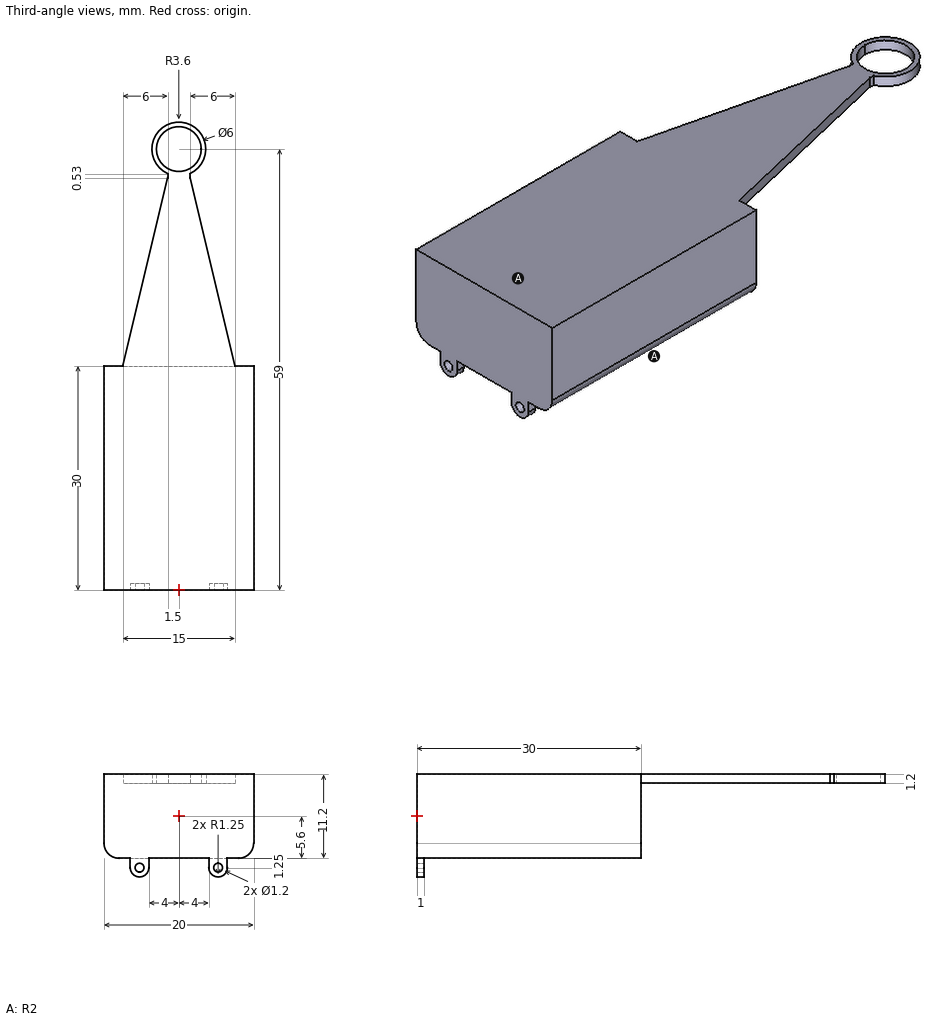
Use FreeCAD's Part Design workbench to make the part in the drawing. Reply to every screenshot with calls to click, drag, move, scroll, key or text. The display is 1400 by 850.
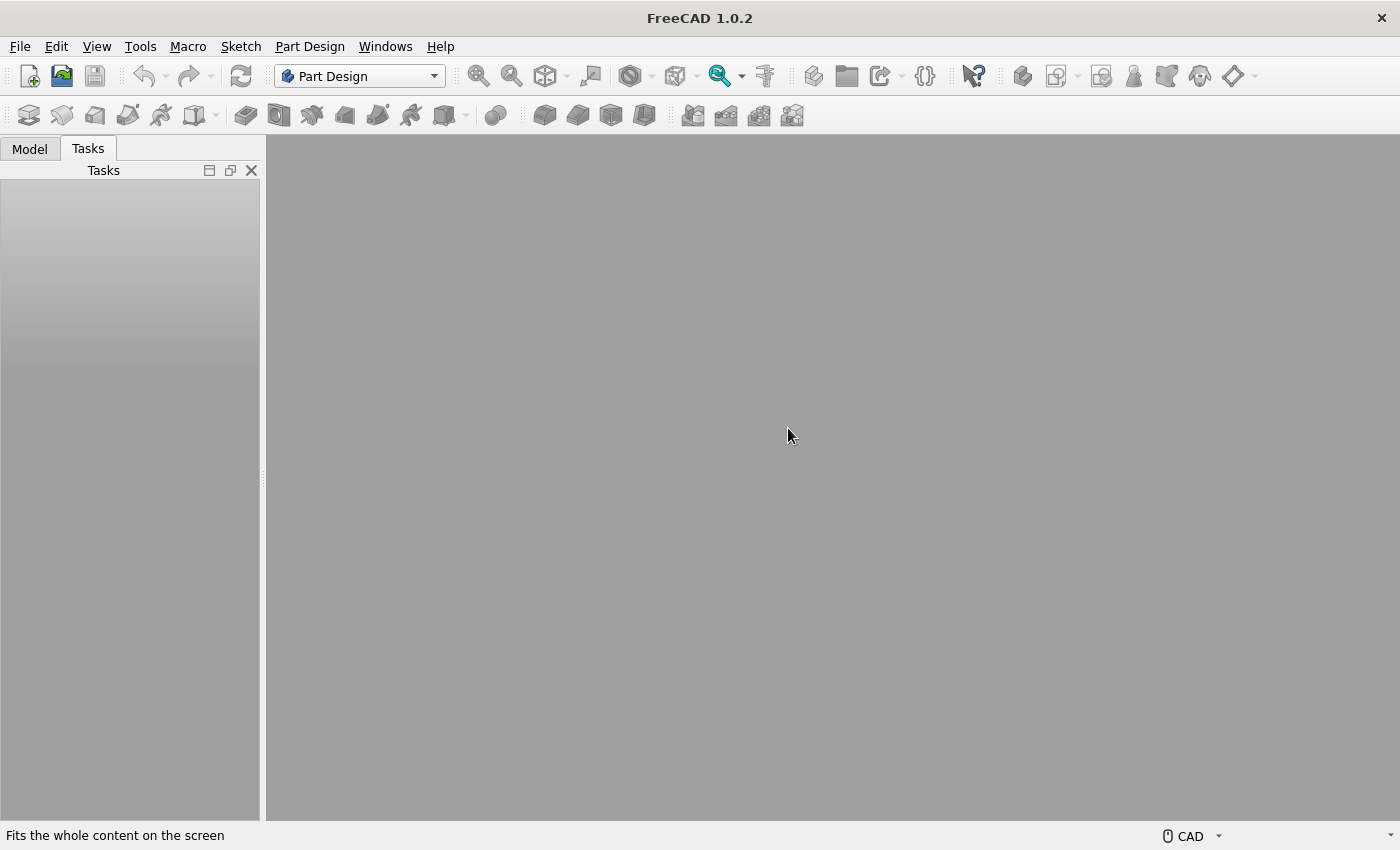
click(29, 76)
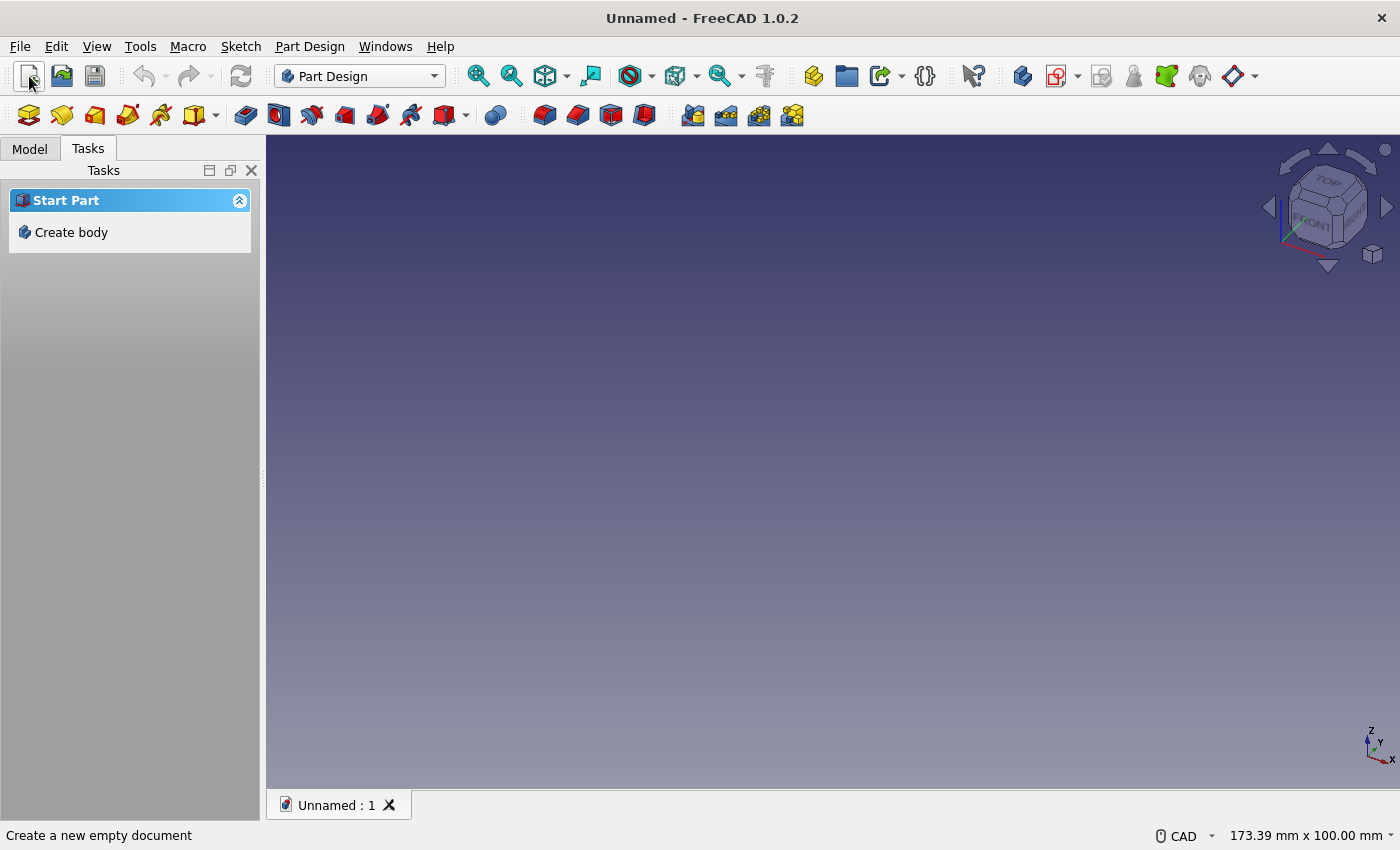
click(1056, 76)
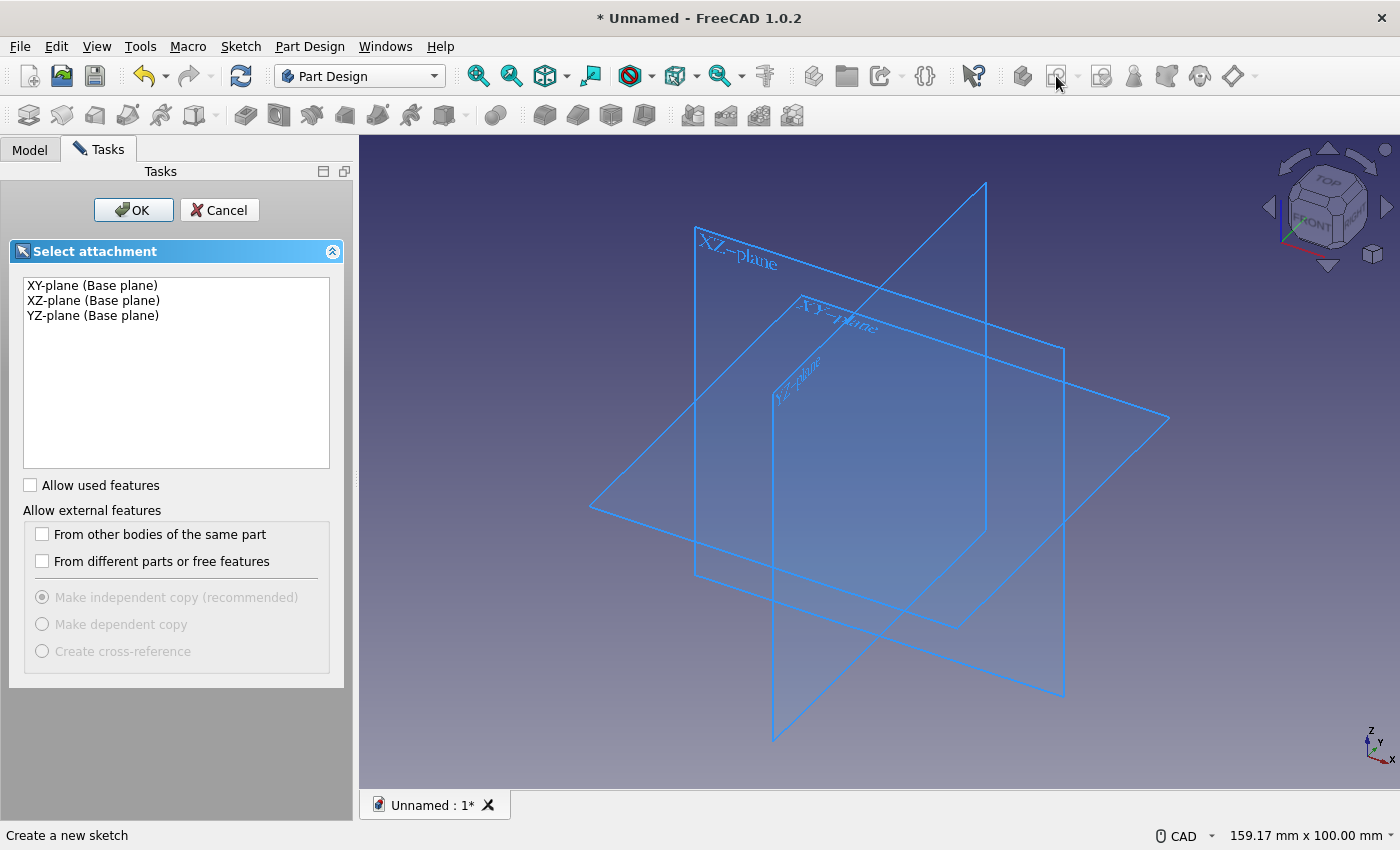
click(84, 300)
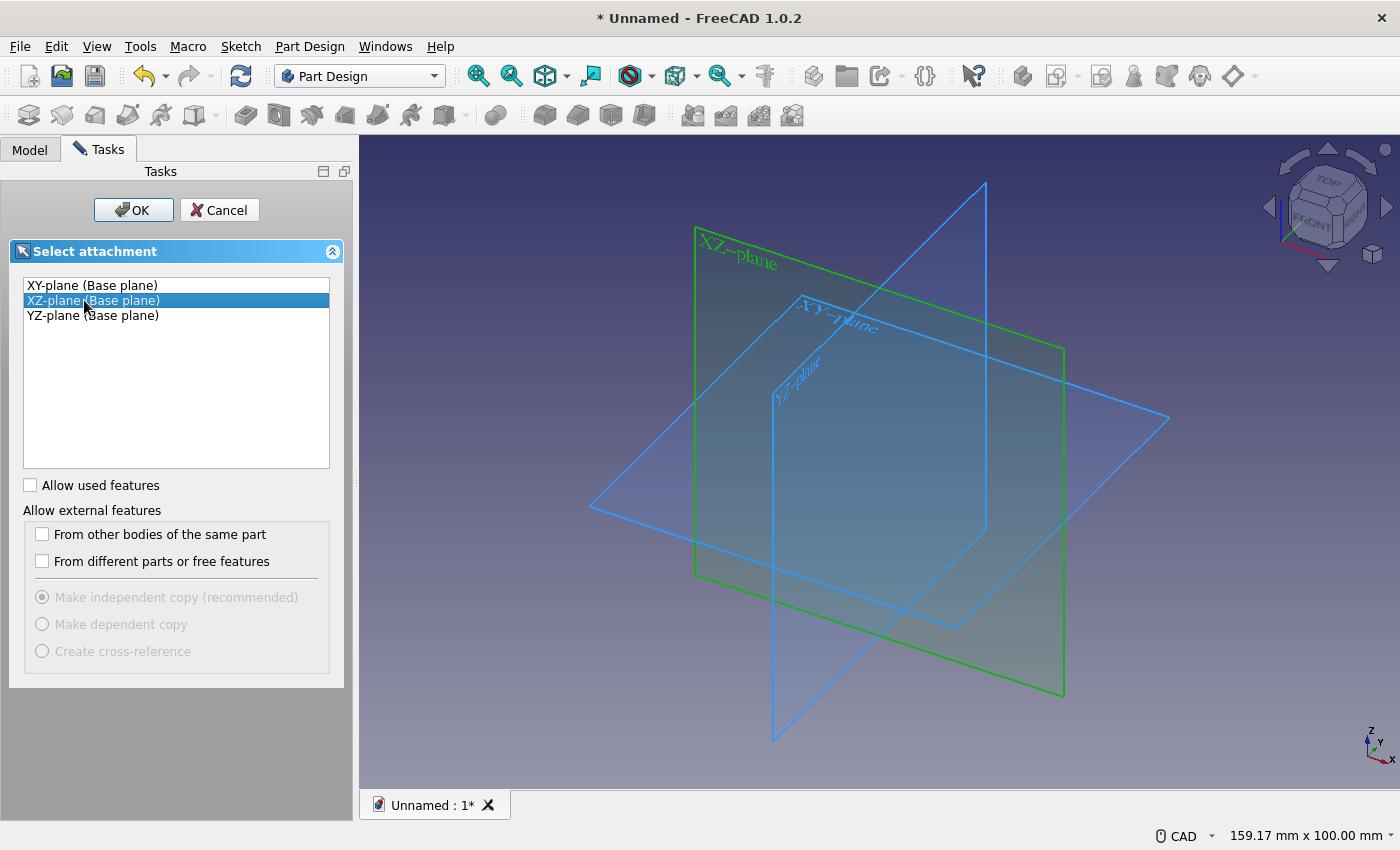
click(134, 210)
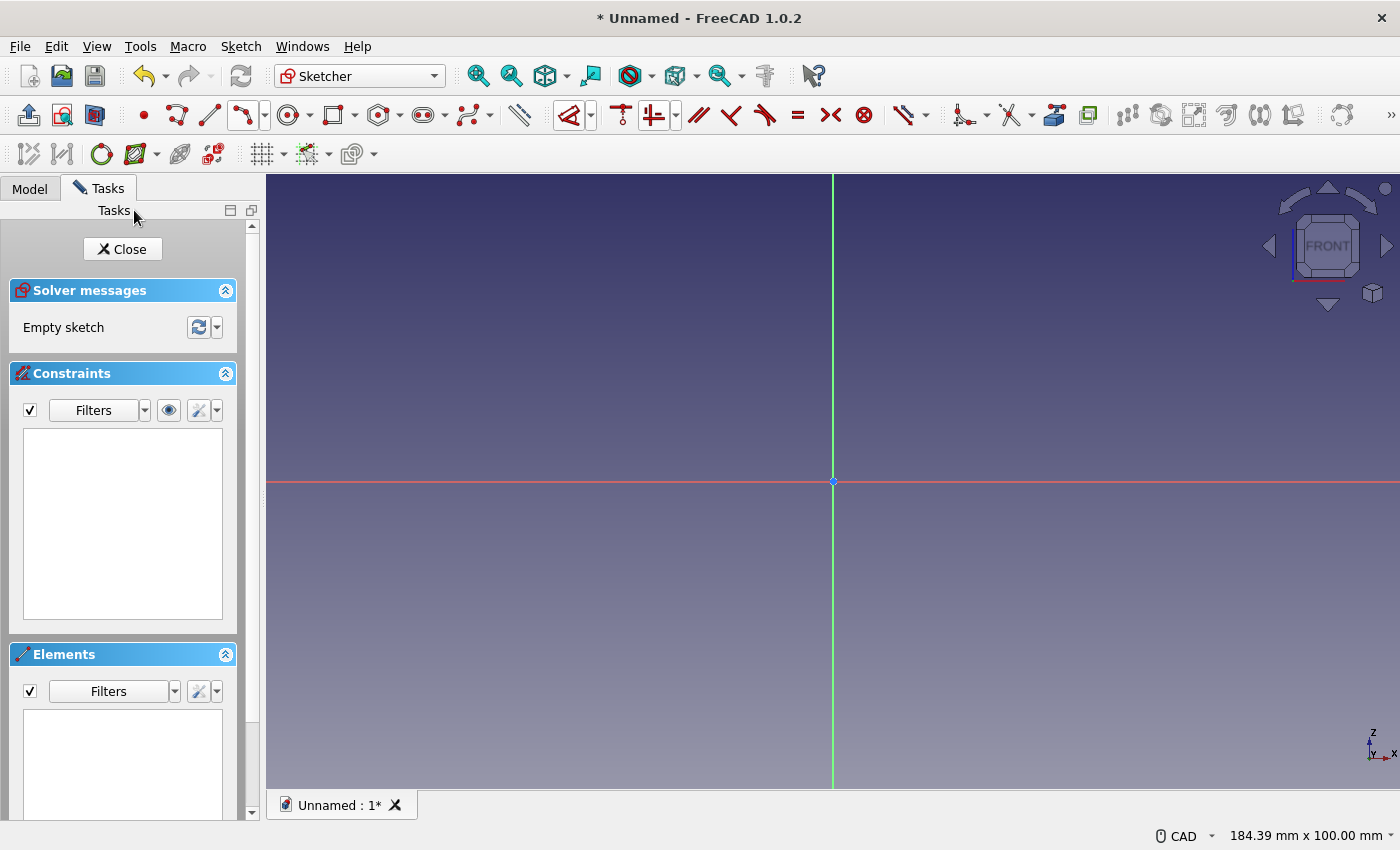
scroll(850, 482, up, 8)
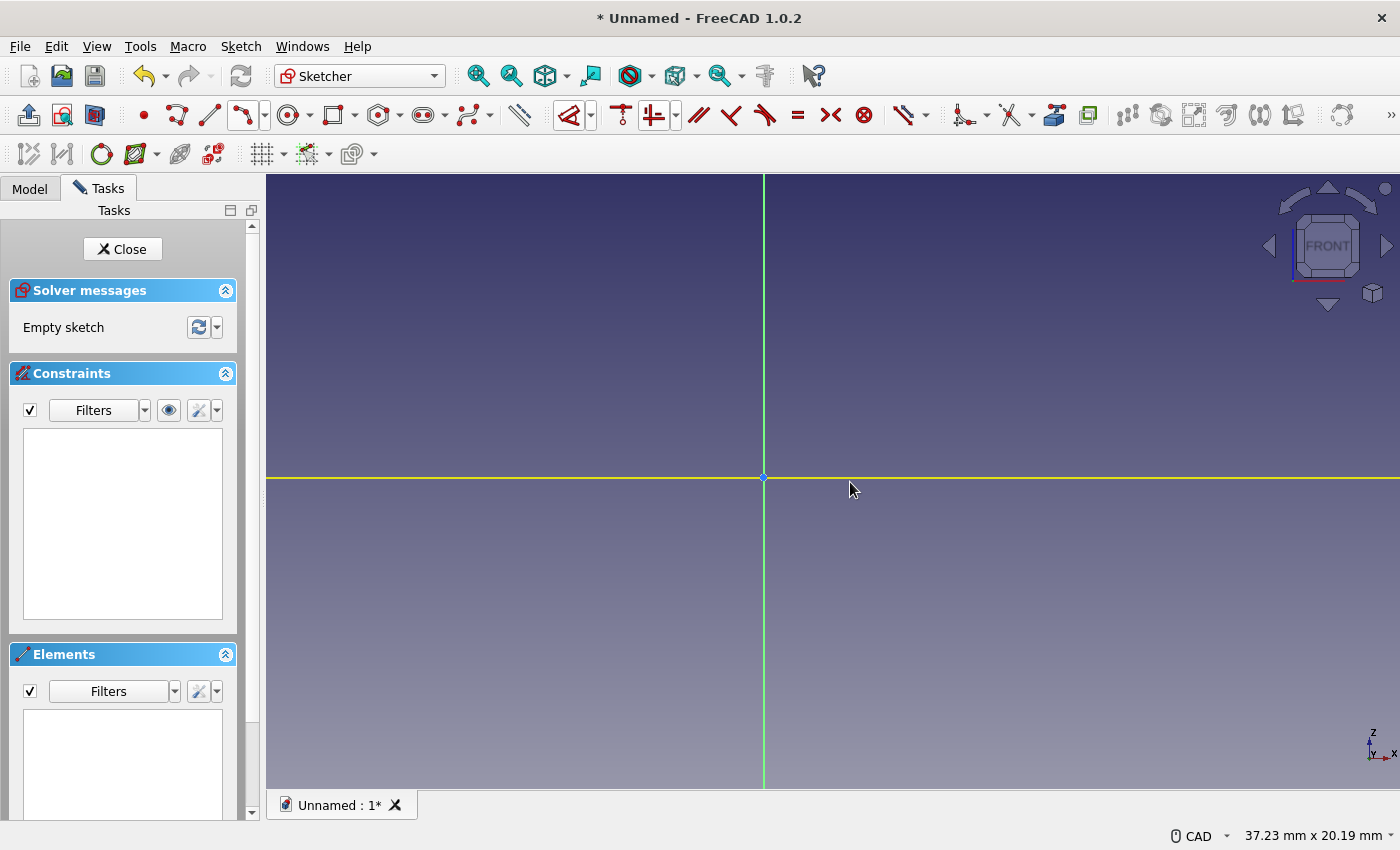
key(g)
key(v)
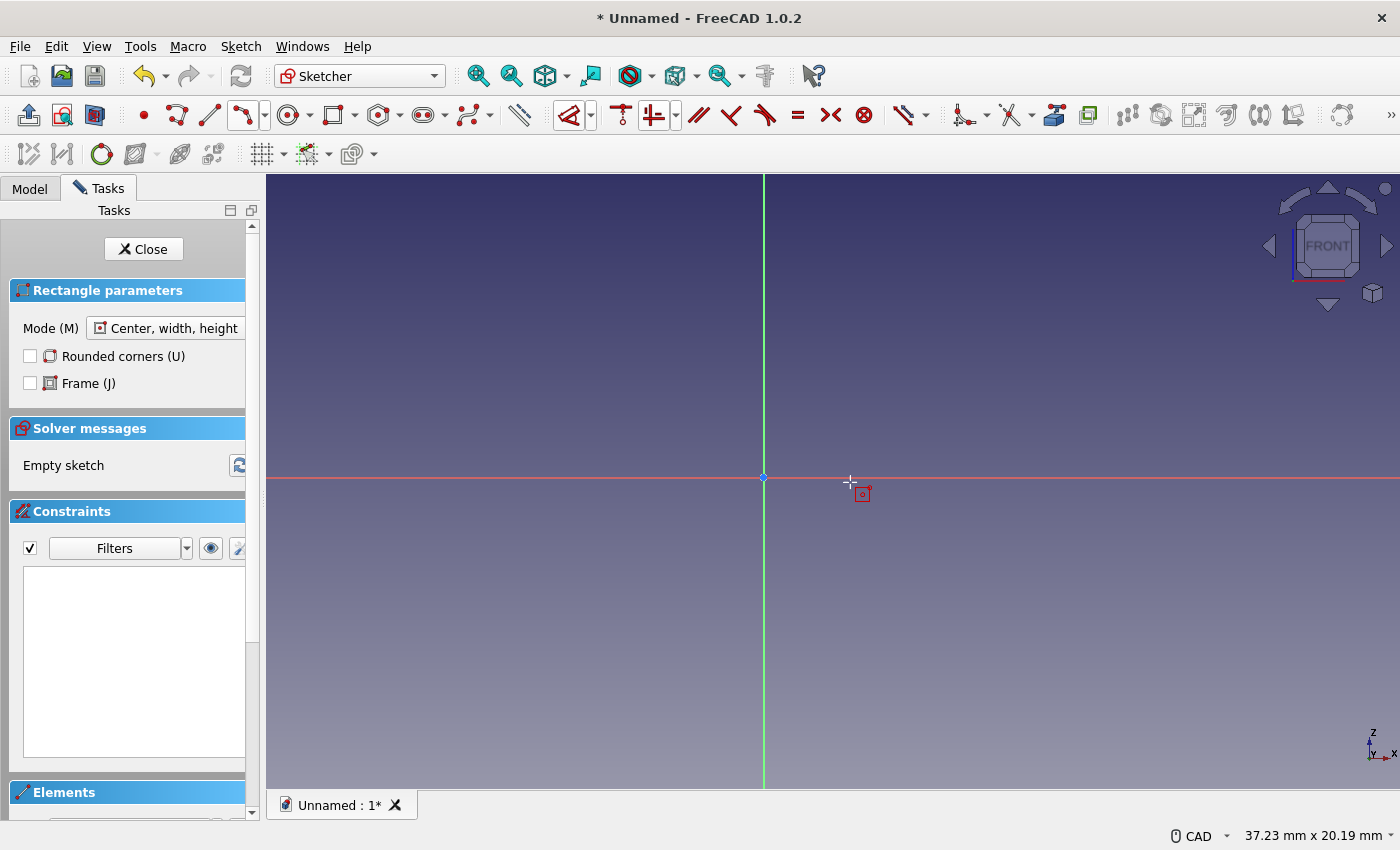
click(764, 478)
click(1068, 307)
key(Escape)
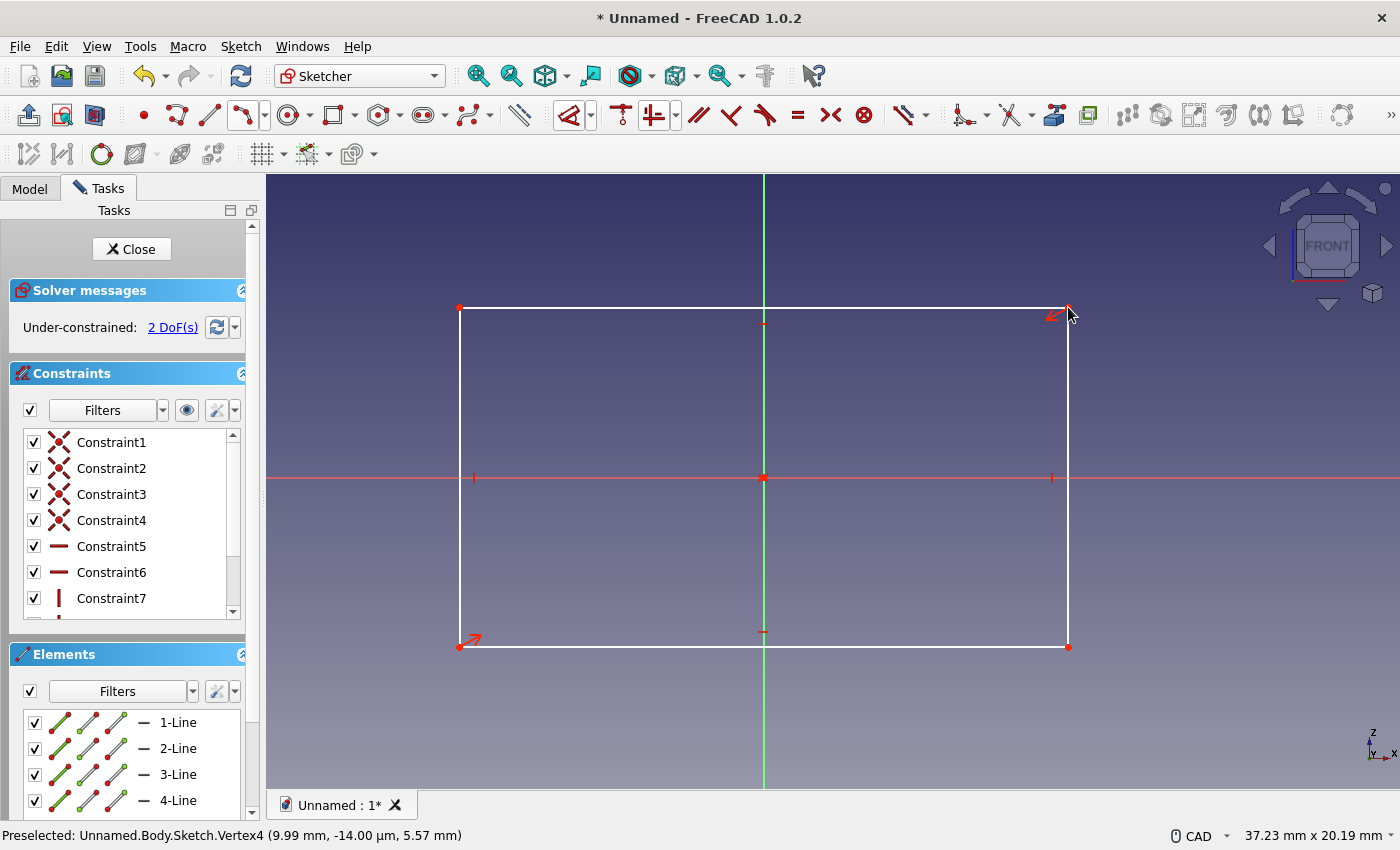
key(d)